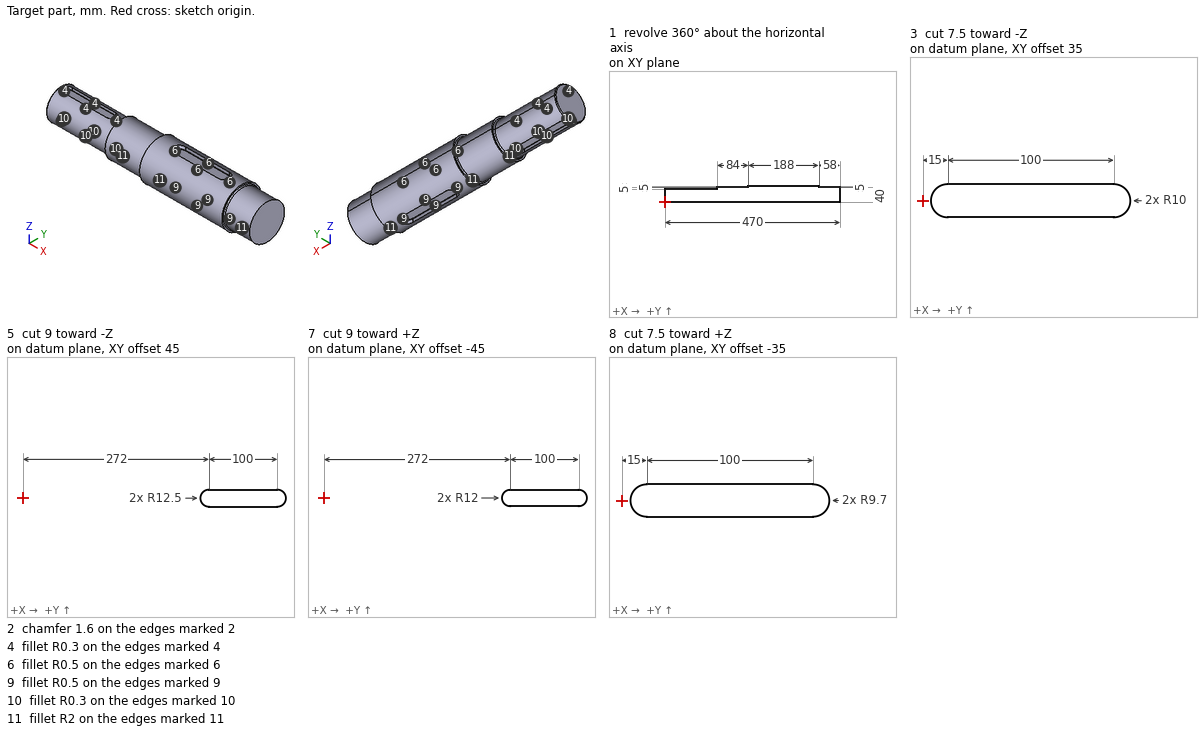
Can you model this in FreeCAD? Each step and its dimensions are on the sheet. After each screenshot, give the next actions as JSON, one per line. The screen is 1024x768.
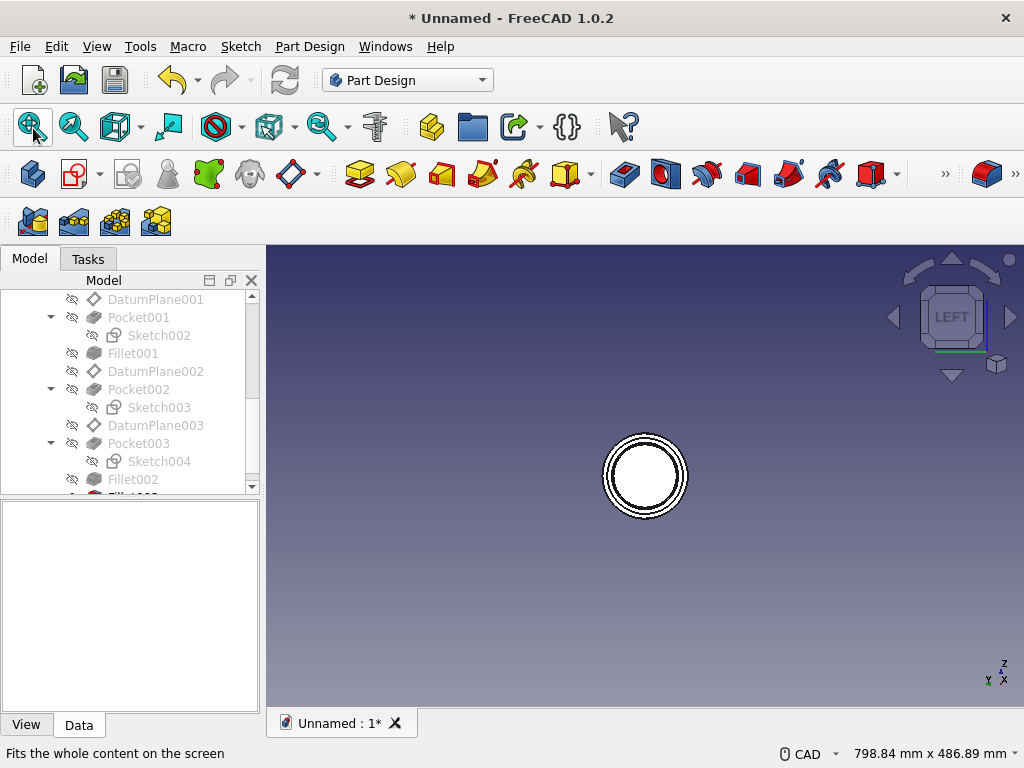
{"action": "key", "text": "v 3"}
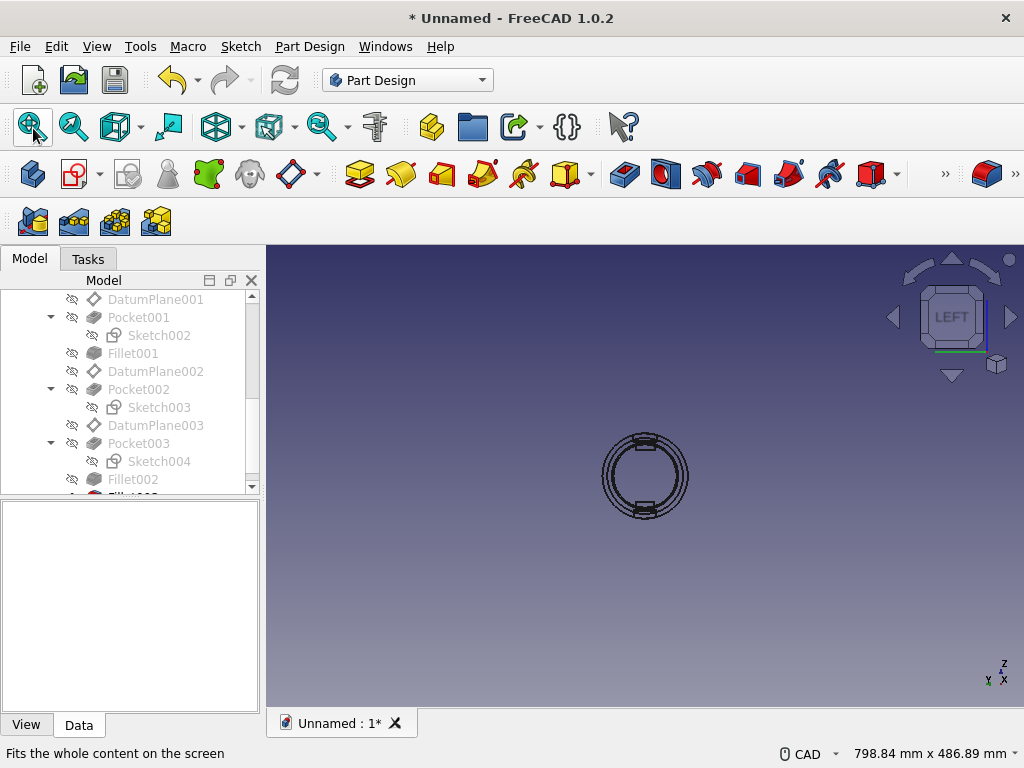
{"action": "key", "text": "0"}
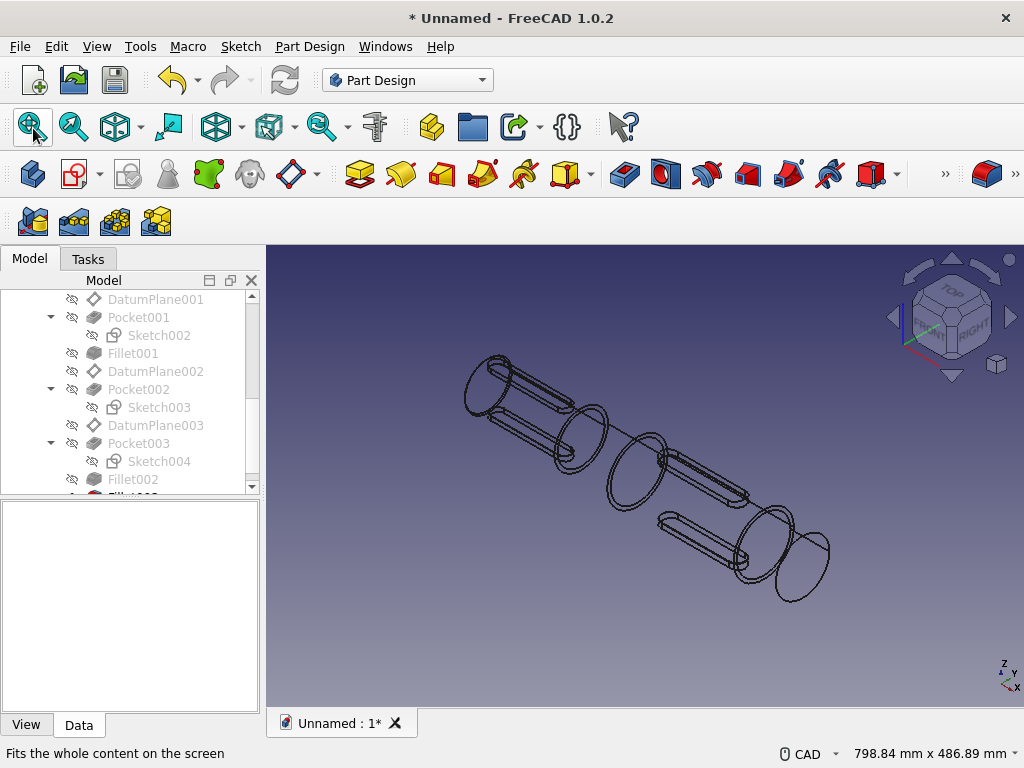
{"action": "left_click", "coordinate": [629, 505]}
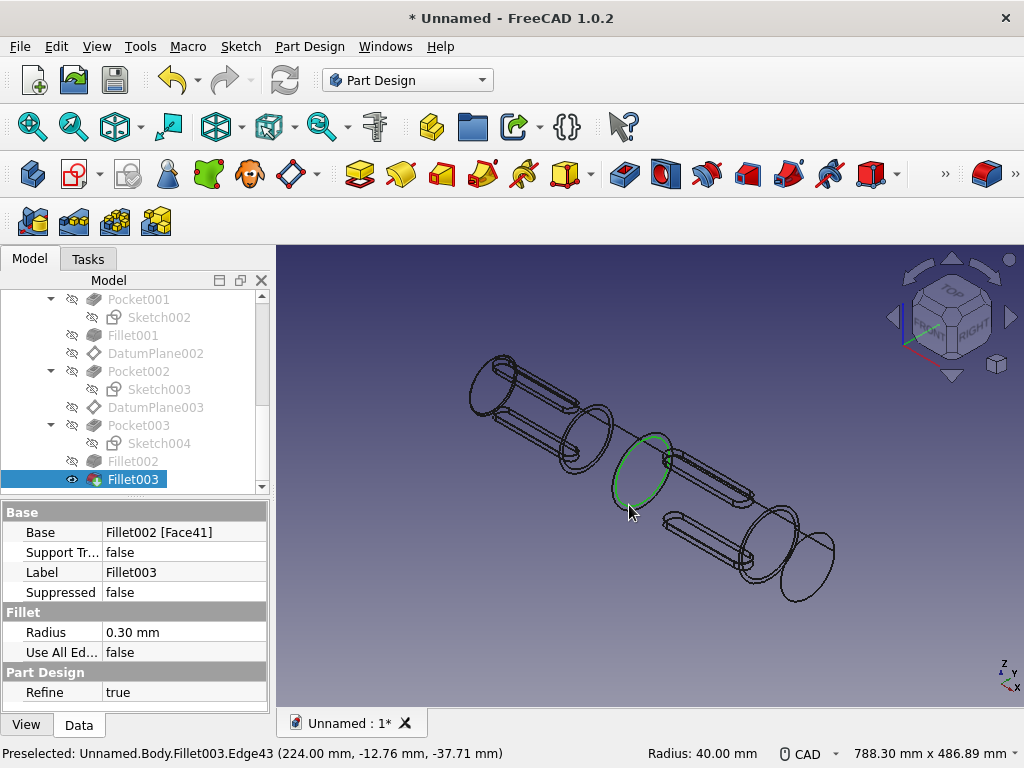
{"action": "left_click", "coordinate": [579, 468], "text": "ctrl"}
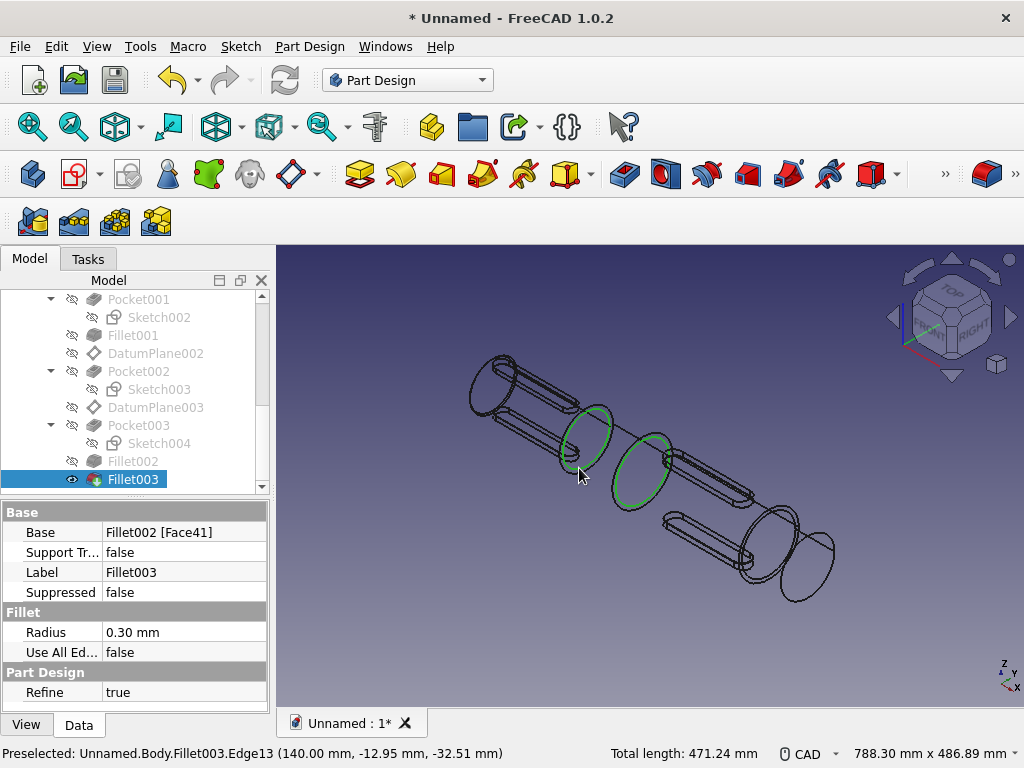
{"action": "left_click", "coordinate": [760, 578], "text": "ctrl"}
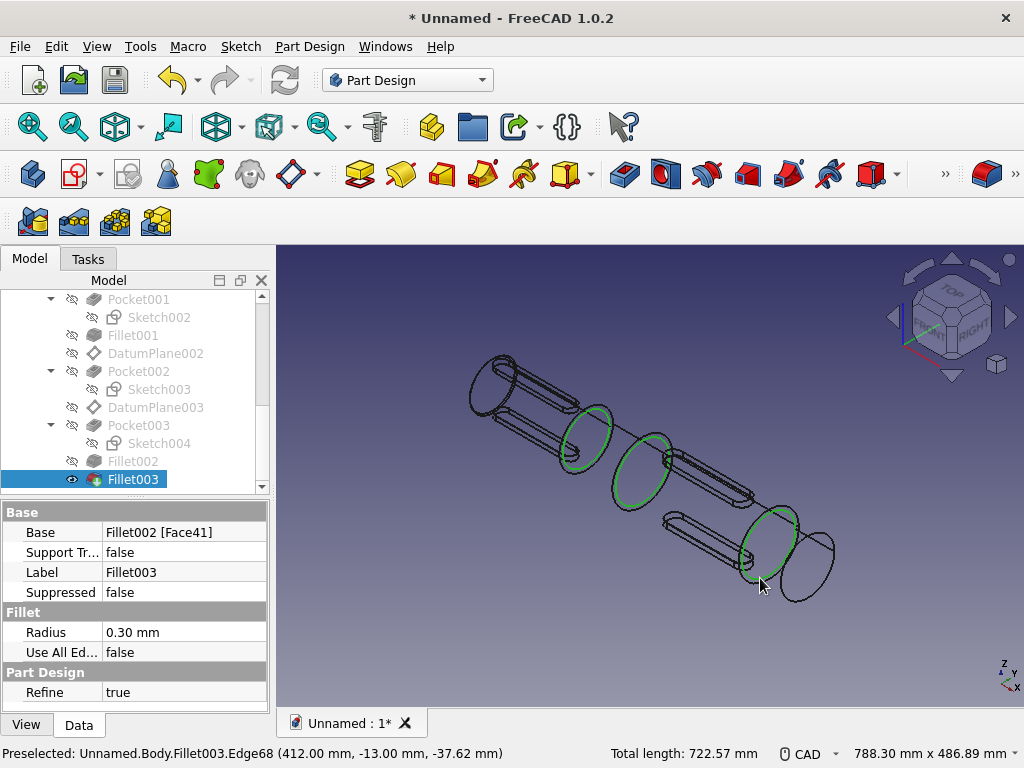
{"action": "key", "text": "v 1"}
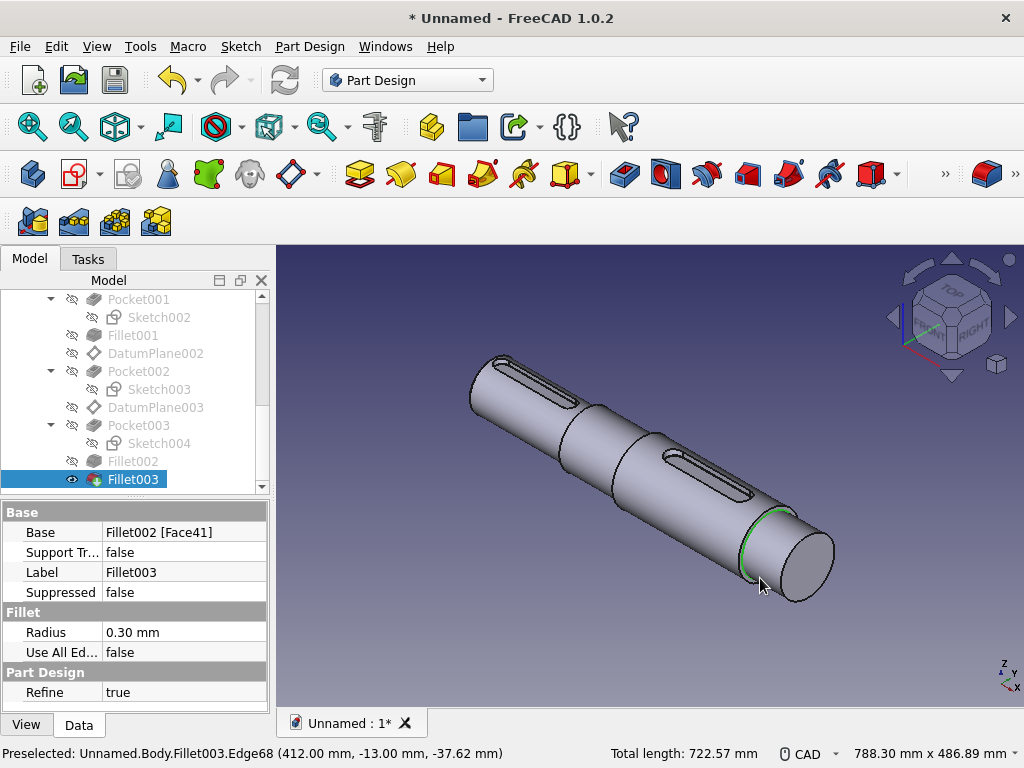
{"action": "left_click", "coordinate": [987, 174]}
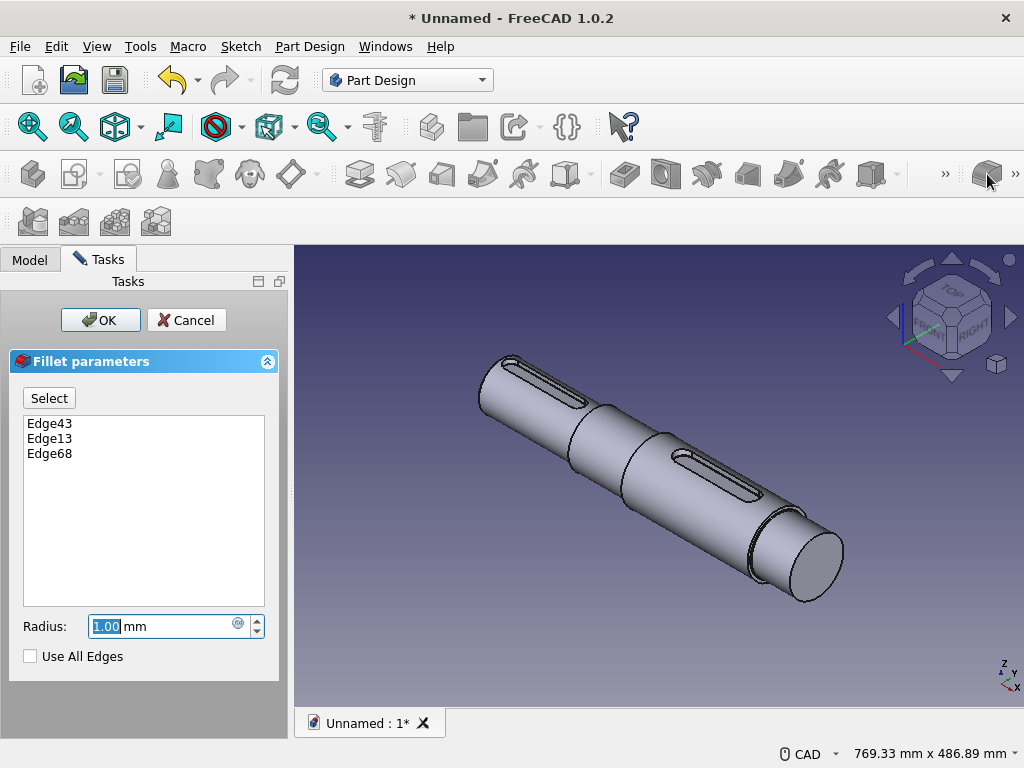
{"action": "type", "text": "2"}
{"action": "key", "text": "Tab"}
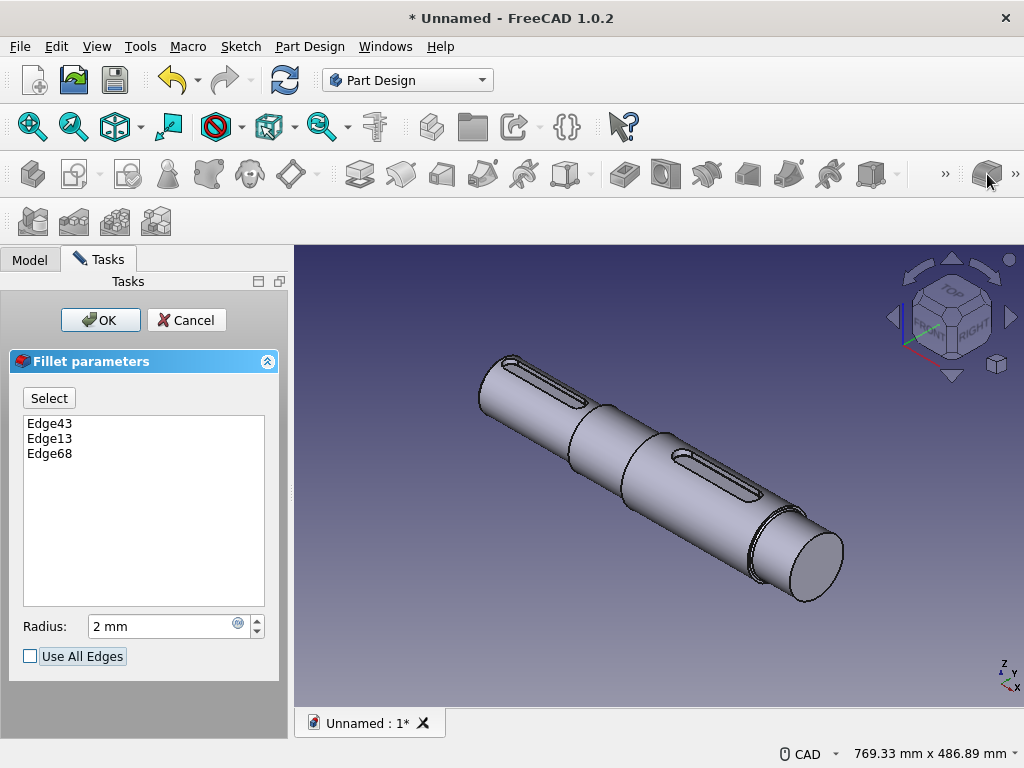
{"action": "left_click", "coordinate": [101, 320]}